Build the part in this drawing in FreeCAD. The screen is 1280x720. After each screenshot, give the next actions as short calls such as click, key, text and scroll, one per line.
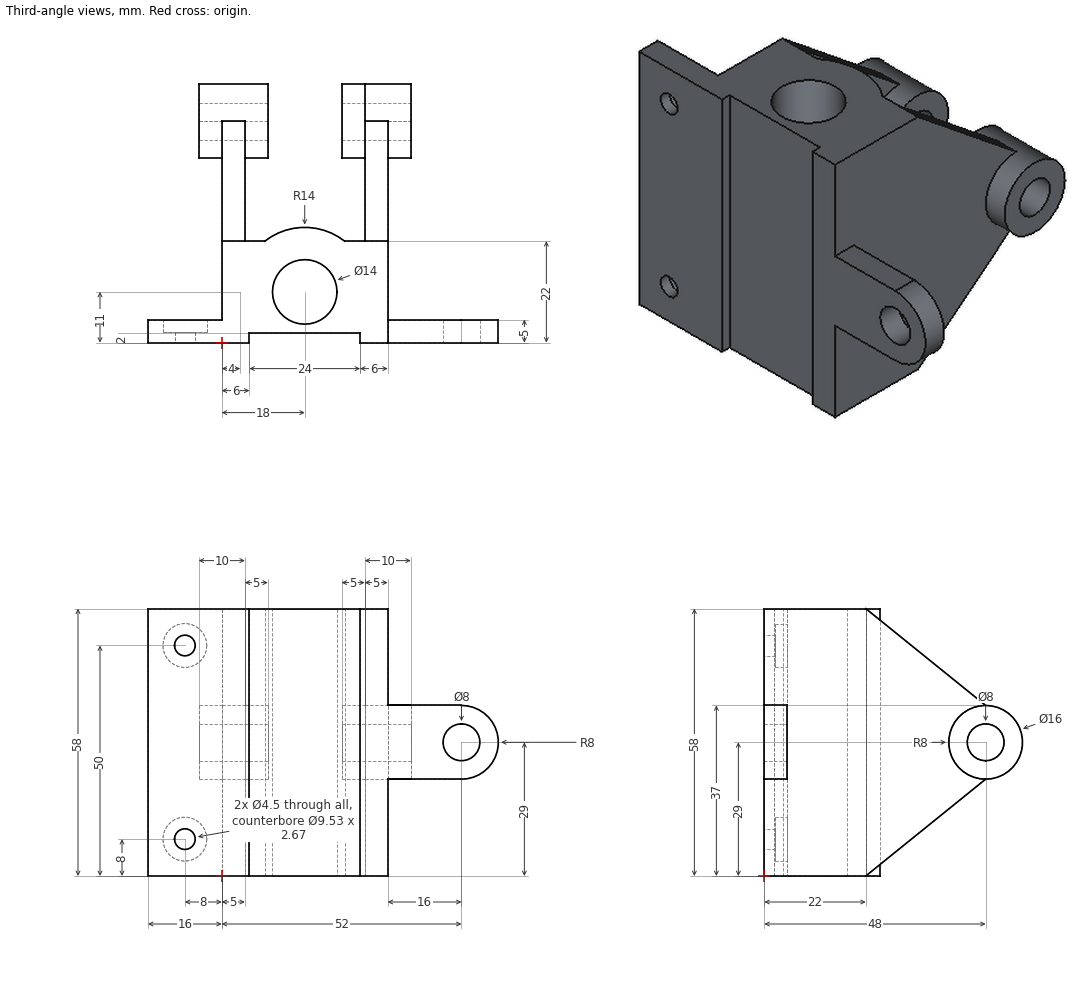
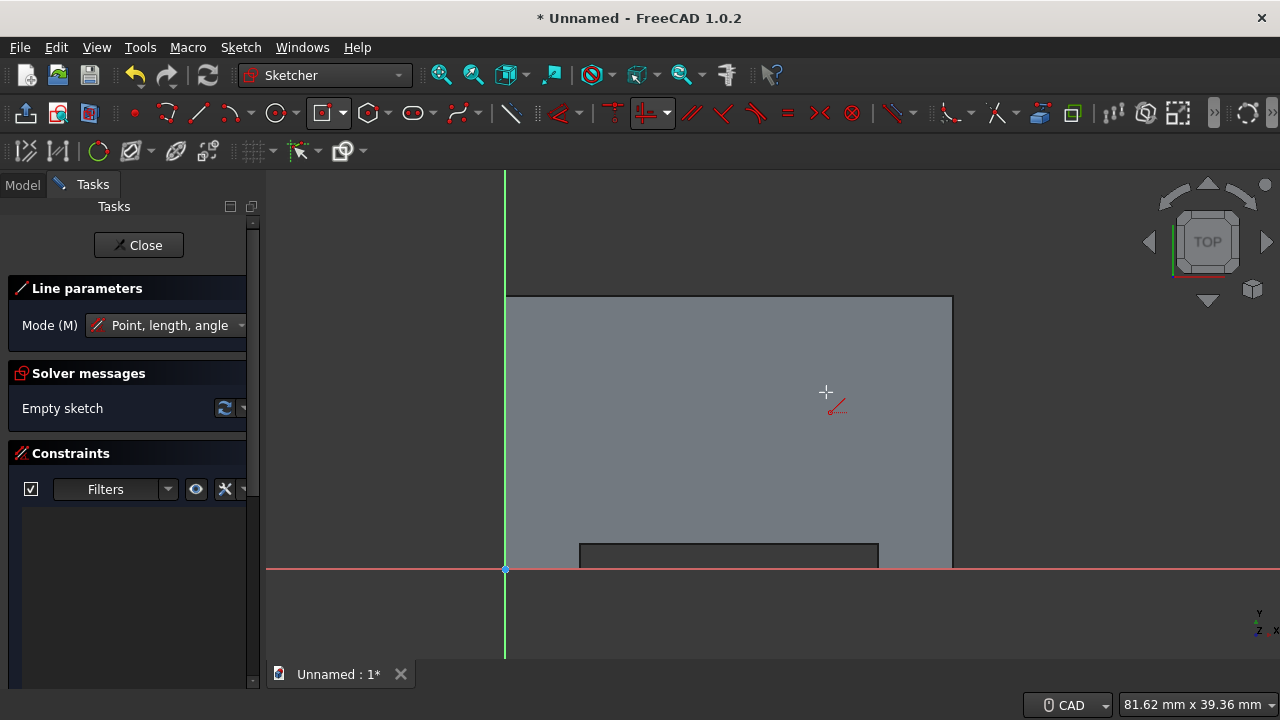
click(555, 433)
click(903, 433)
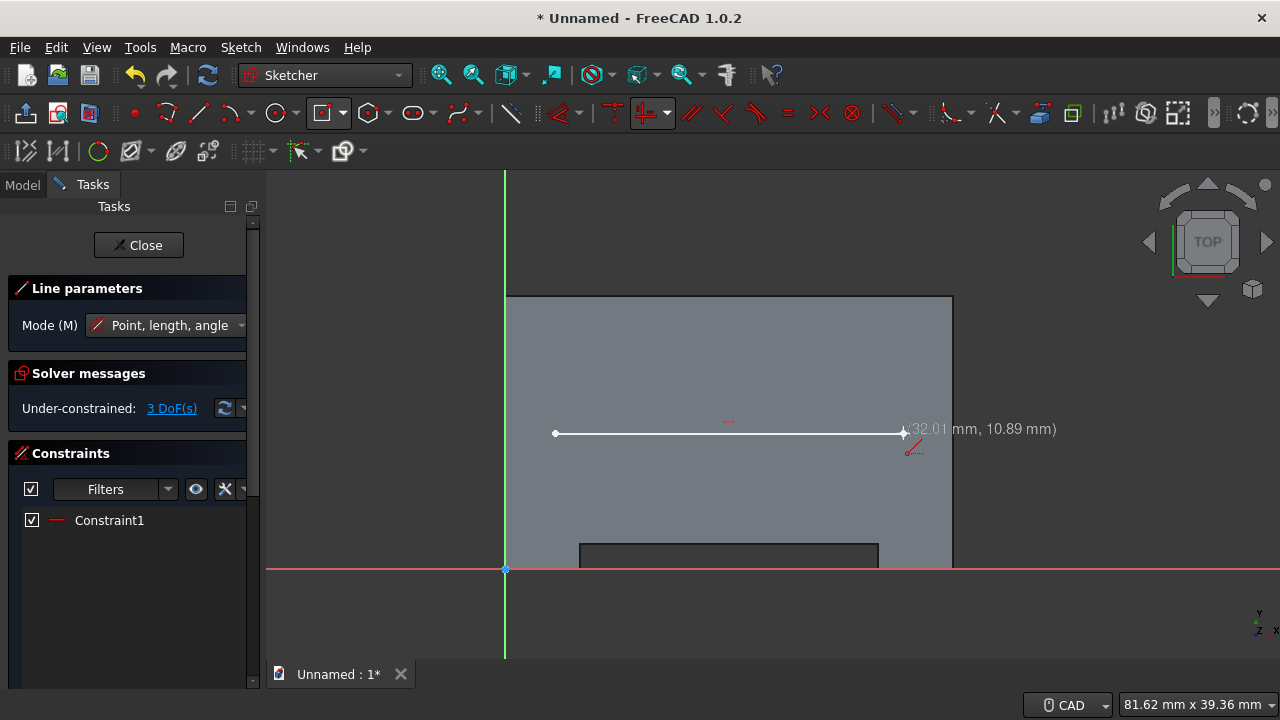
key(g)
key(3)
key(a)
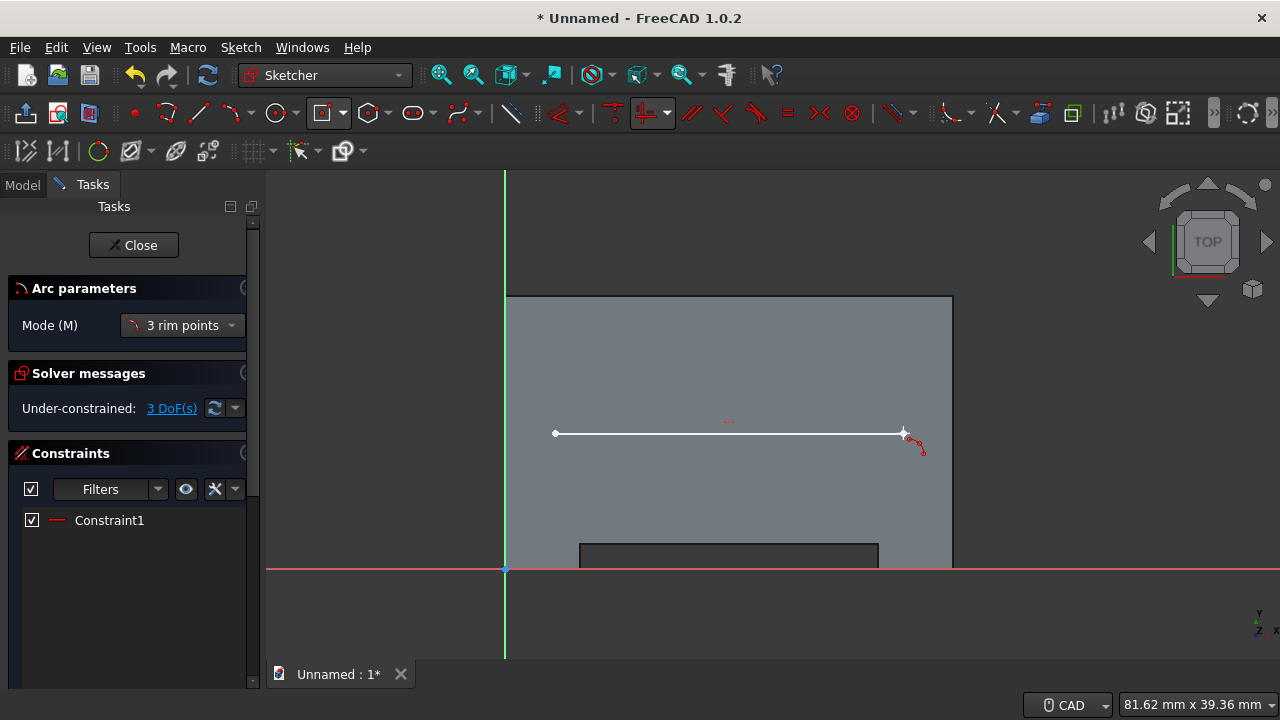
click(903, 434)
click(555, 434)
click(729, 259)
key(Escape)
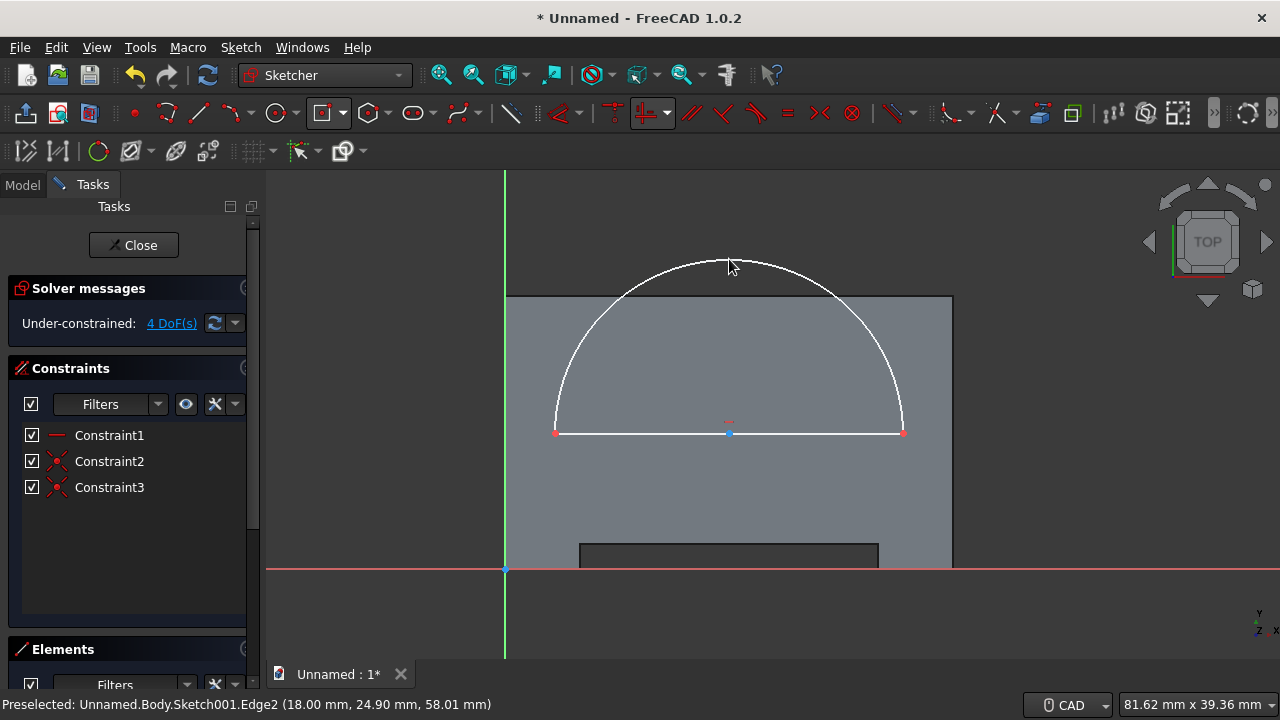
key(d)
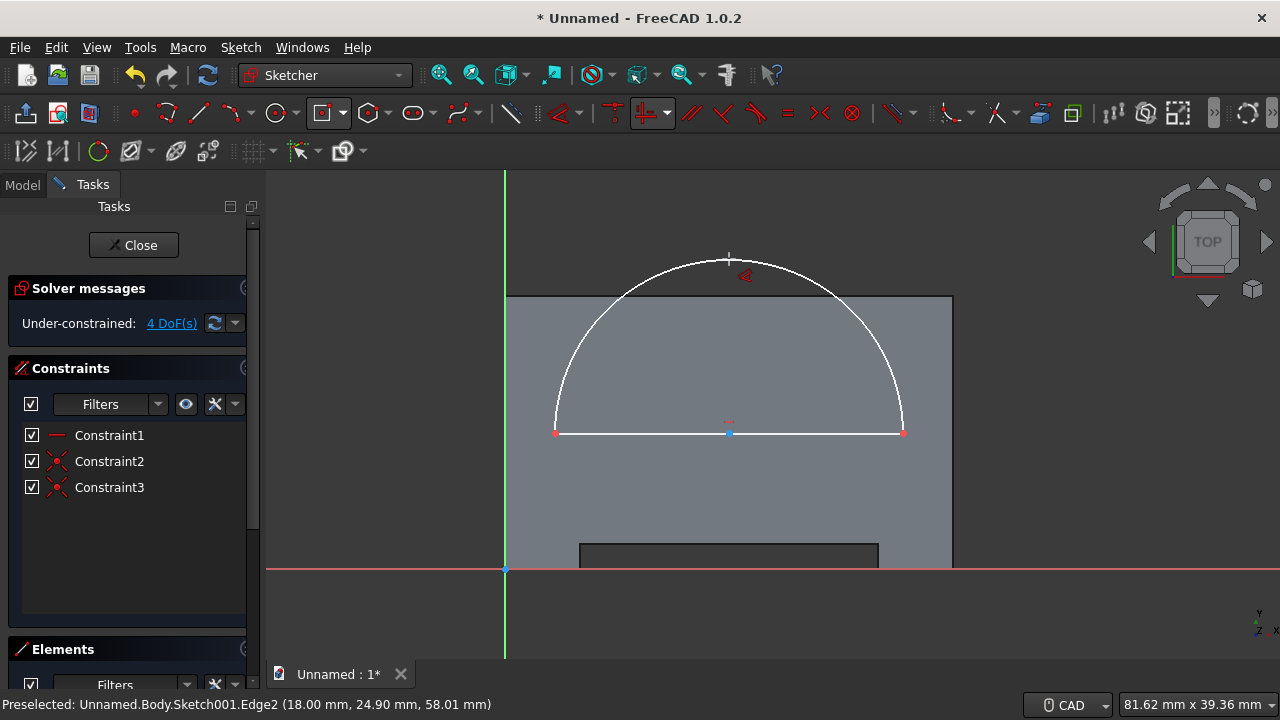
click(831, 293)
click(850, 267)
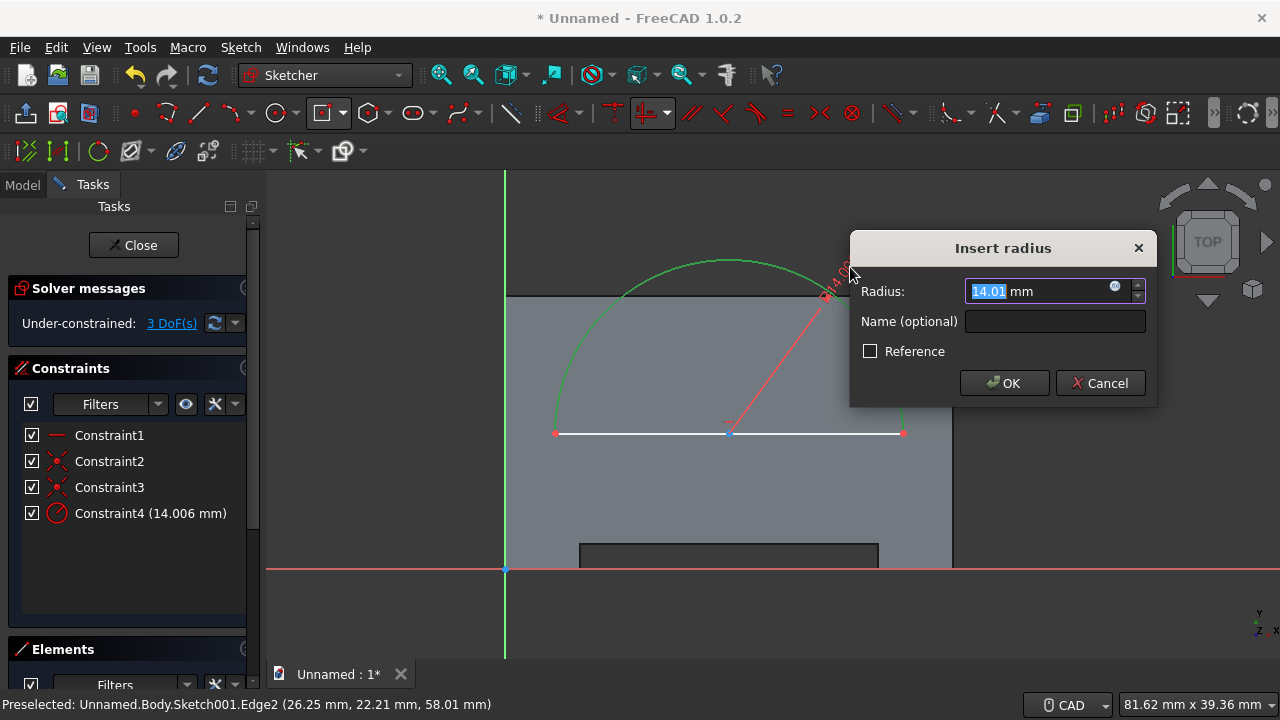
text(14)
key(Return)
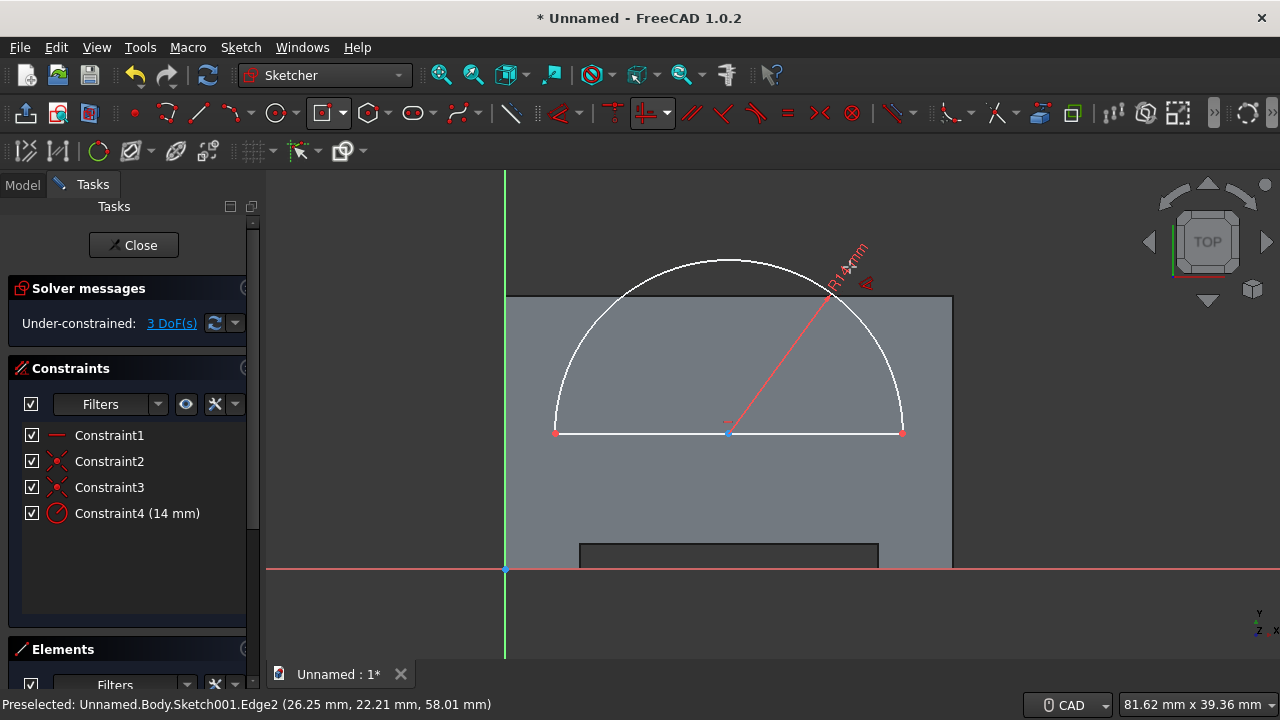
click(555, 434)
click(530, 603)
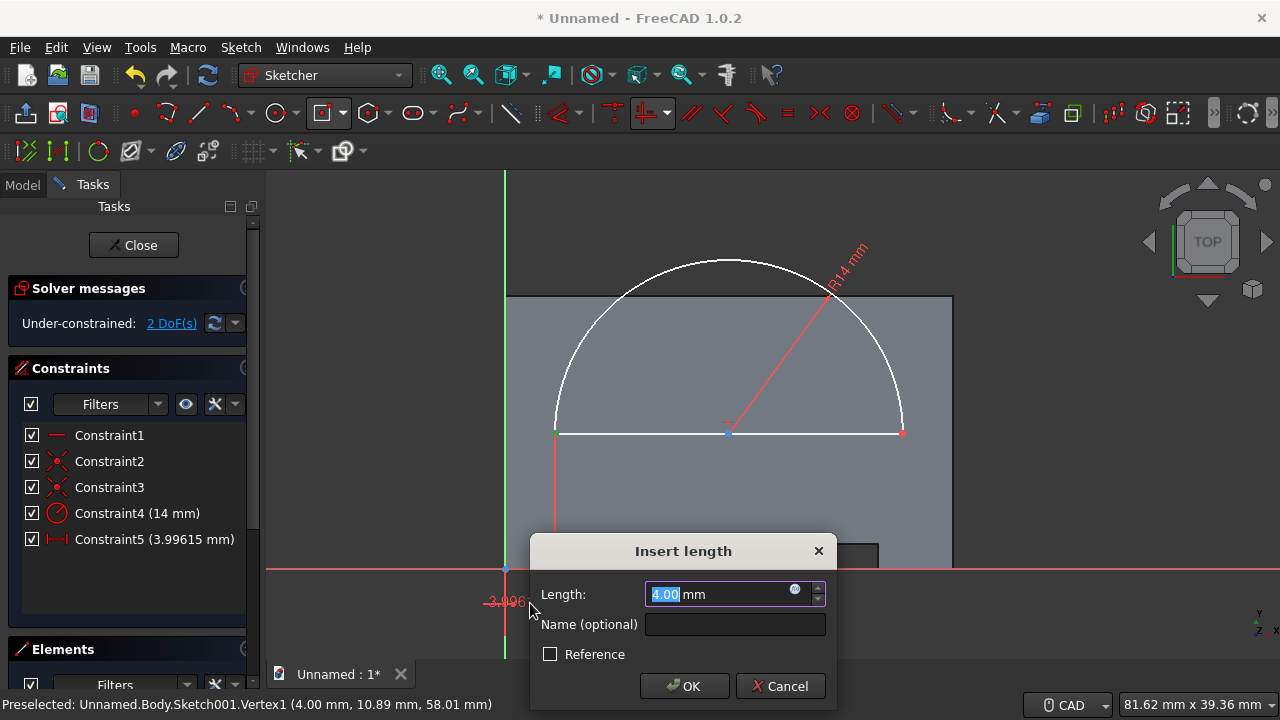
text(4)
key(Return)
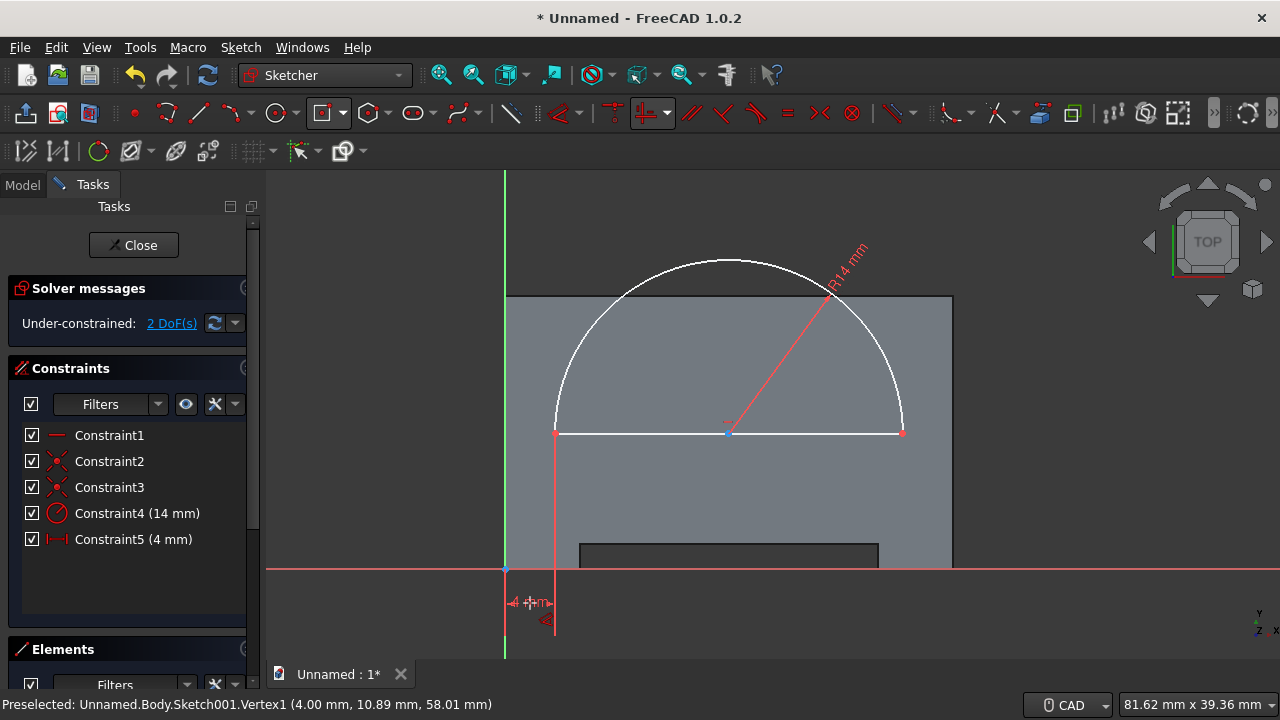
click(555, 434)
click(471, 502)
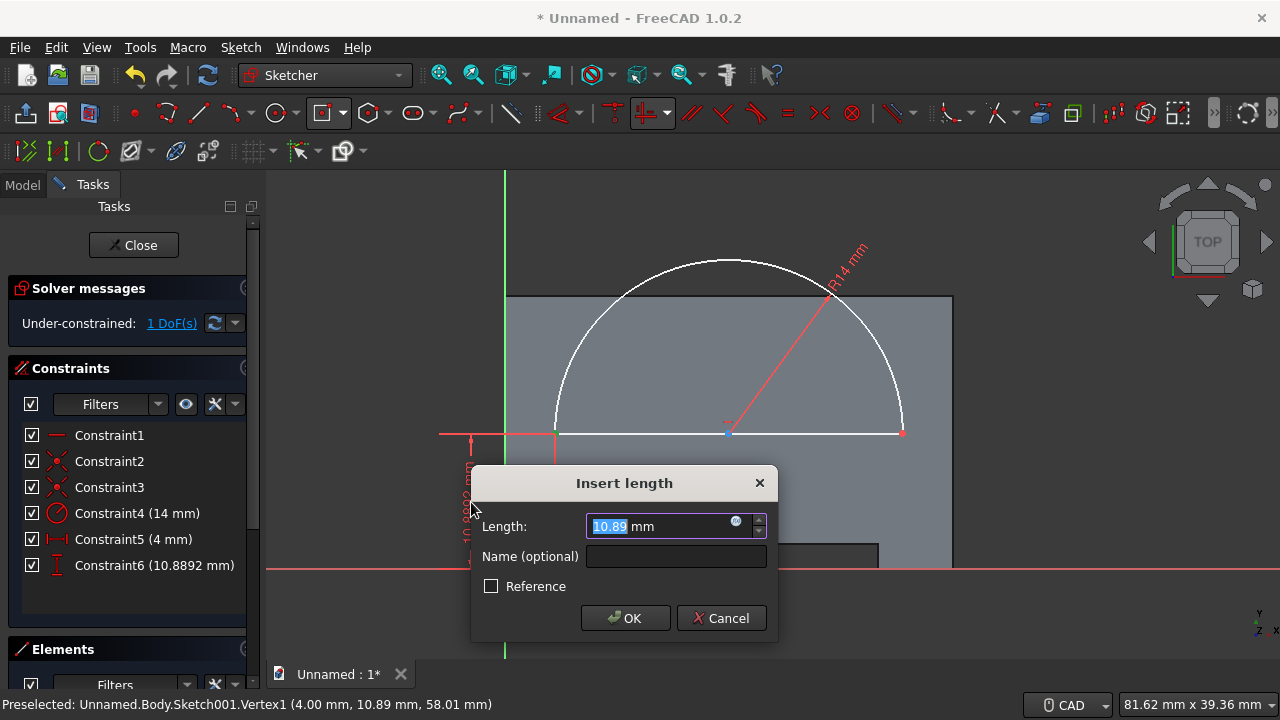
text(11)
key(Return)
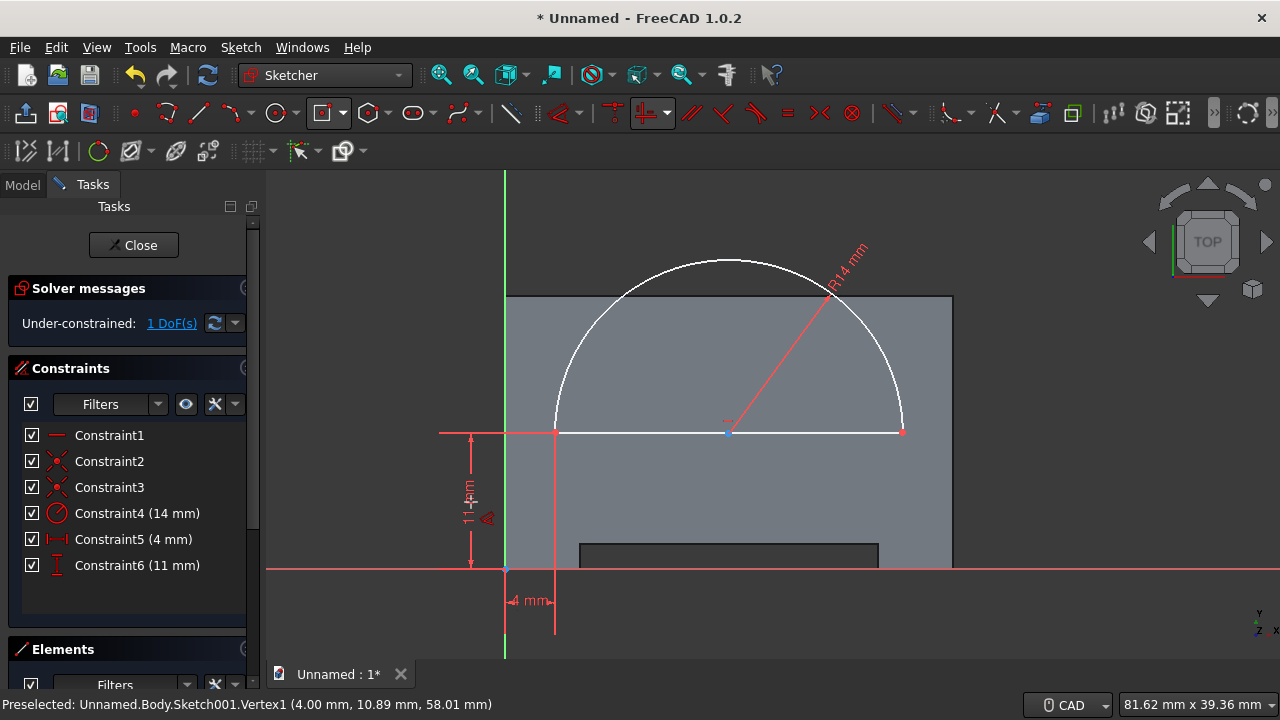
click(729, 434)
click(471, 471)